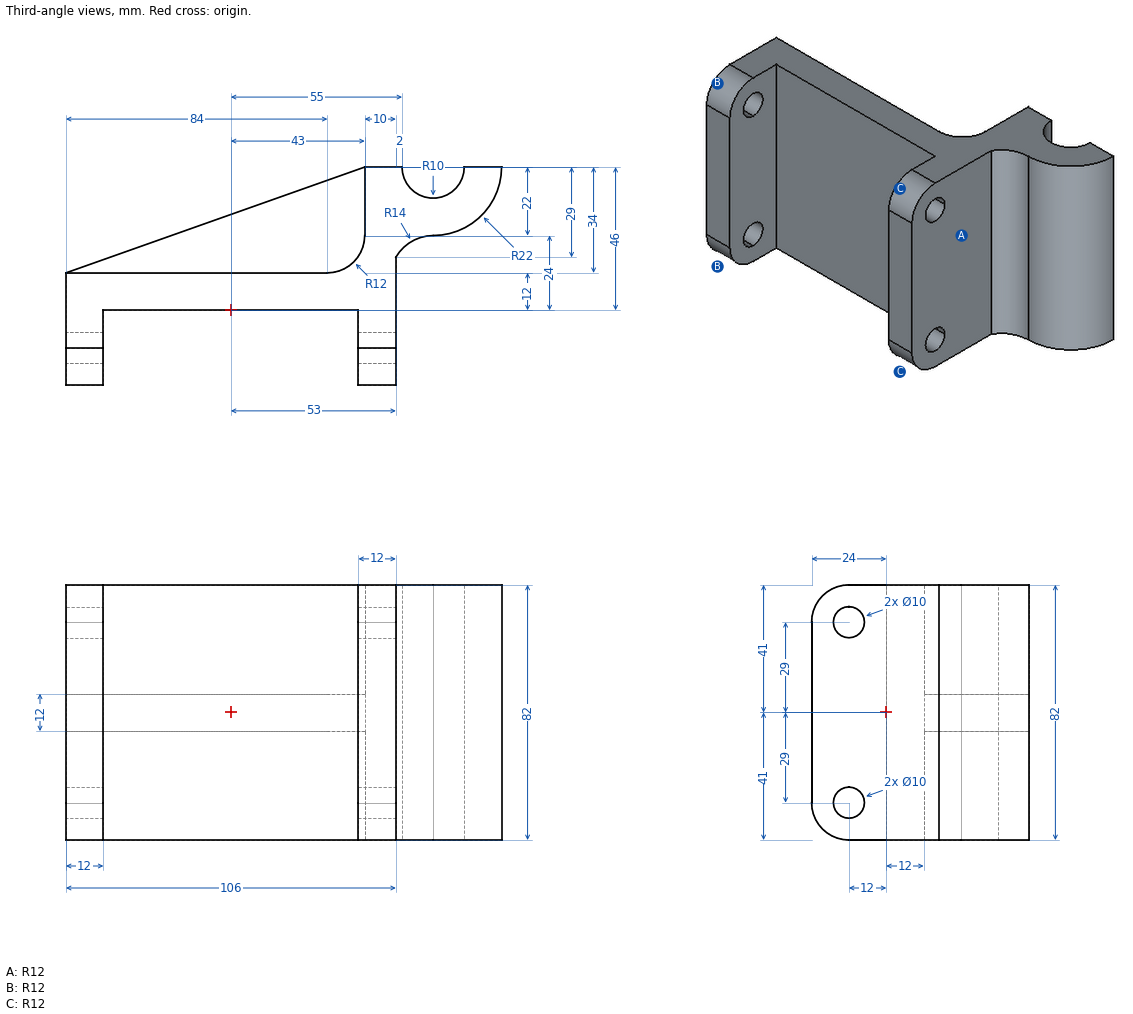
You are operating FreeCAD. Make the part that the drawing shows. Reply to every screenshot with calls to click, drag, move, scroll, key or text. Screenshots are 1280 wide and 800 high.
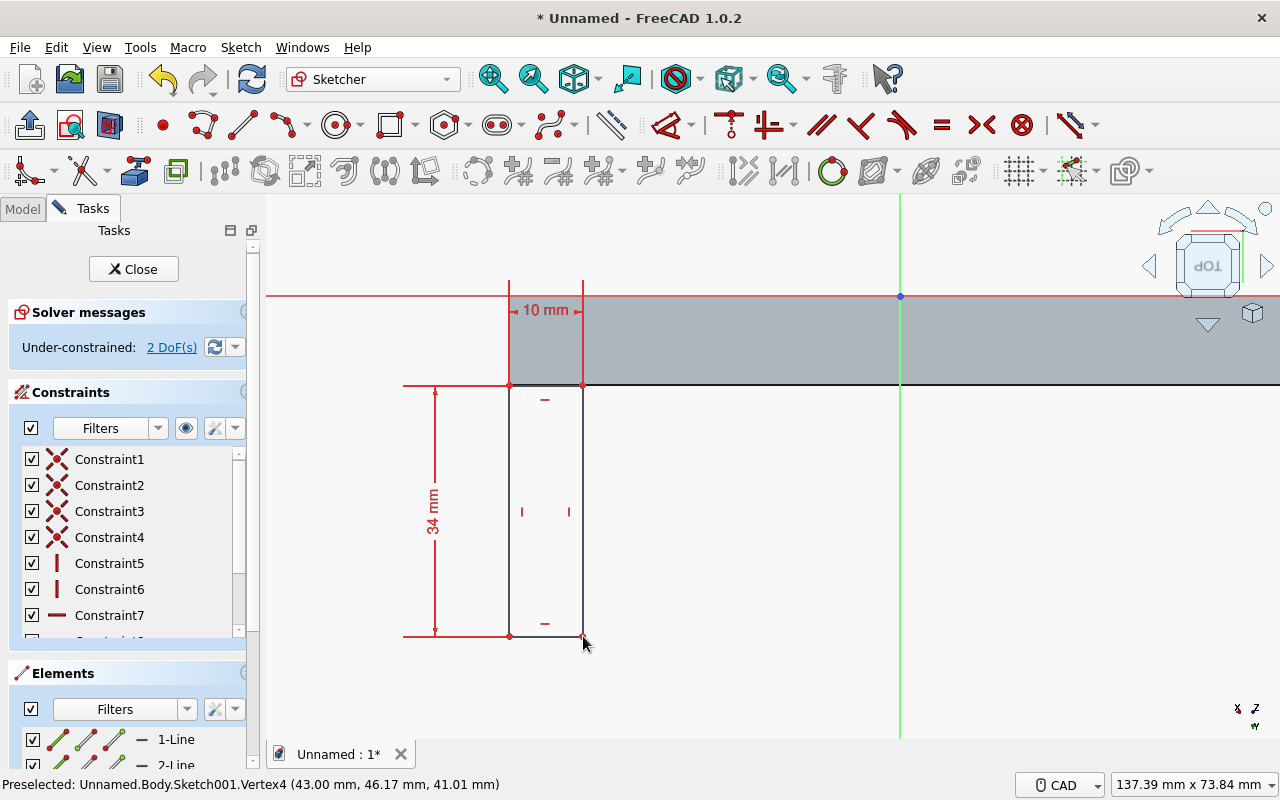
key(d)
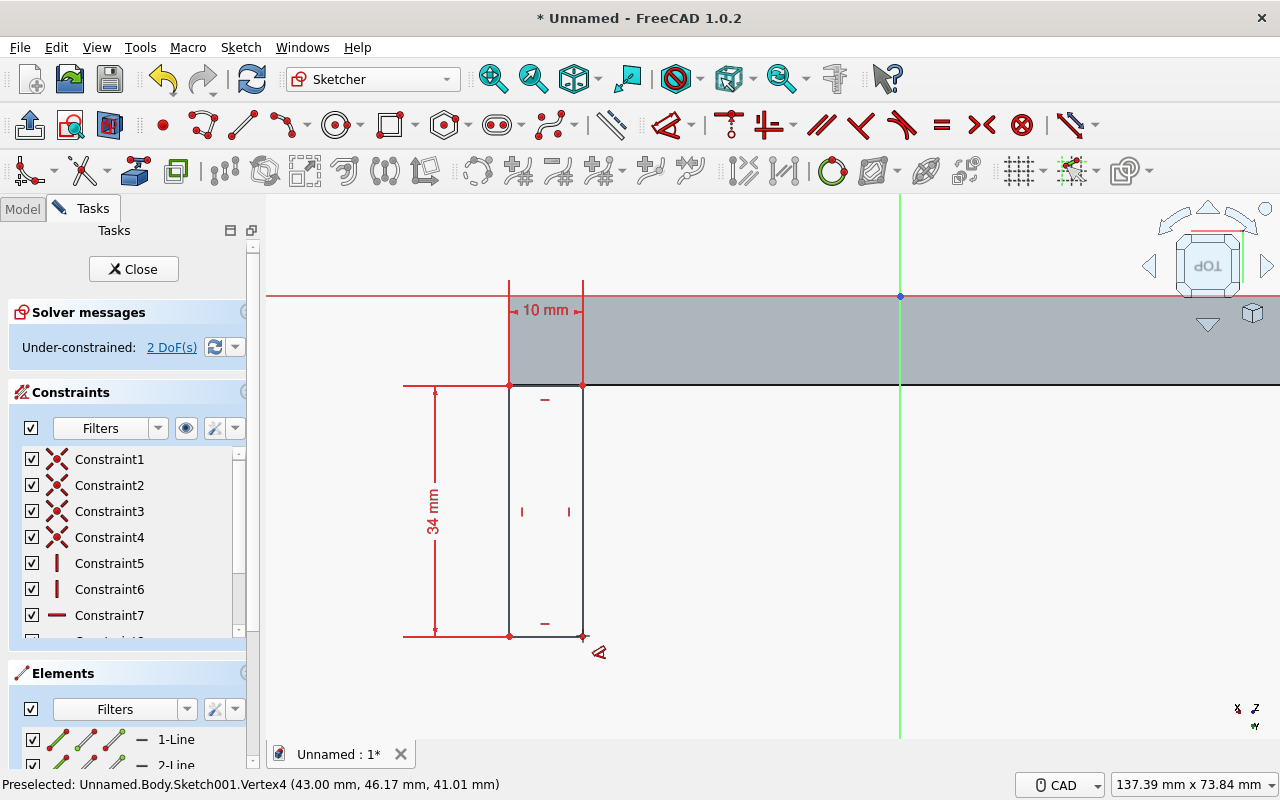
click(509, 386)
click(705, 262)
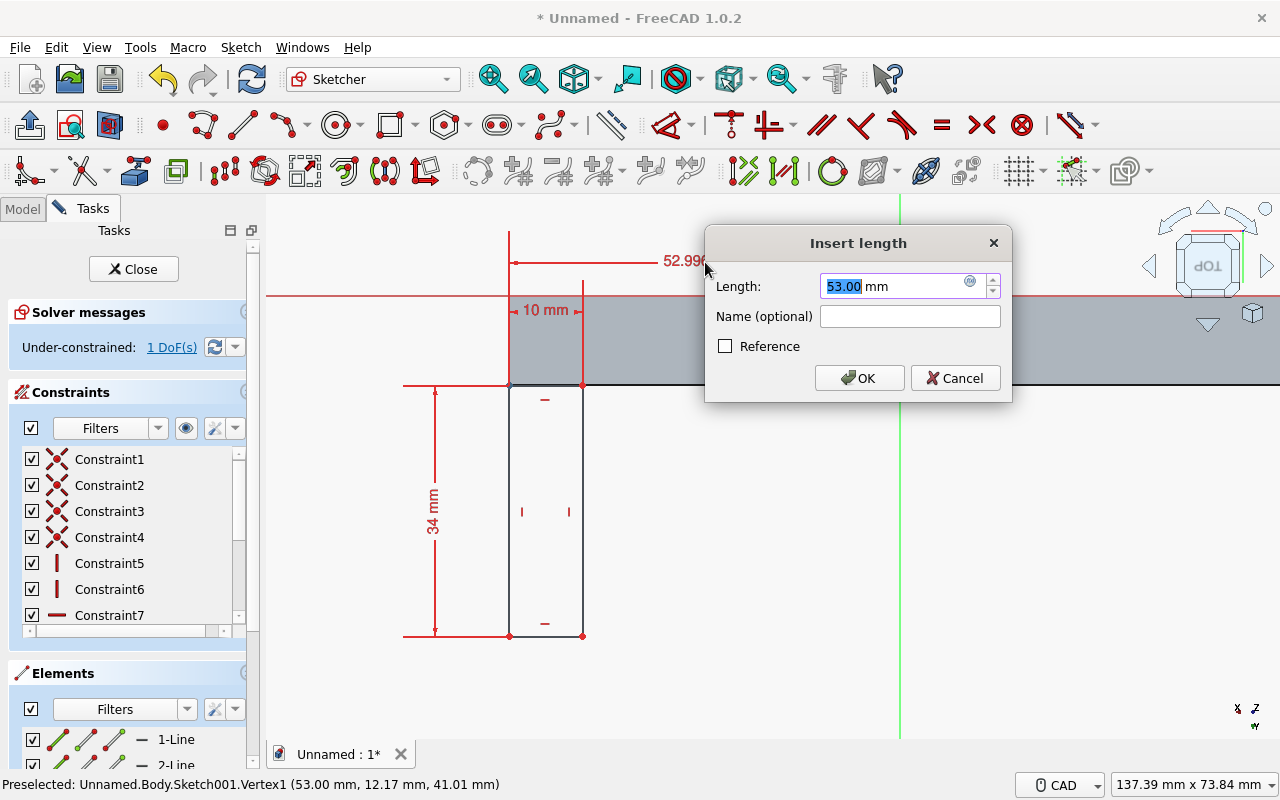
text(53)
key(Return)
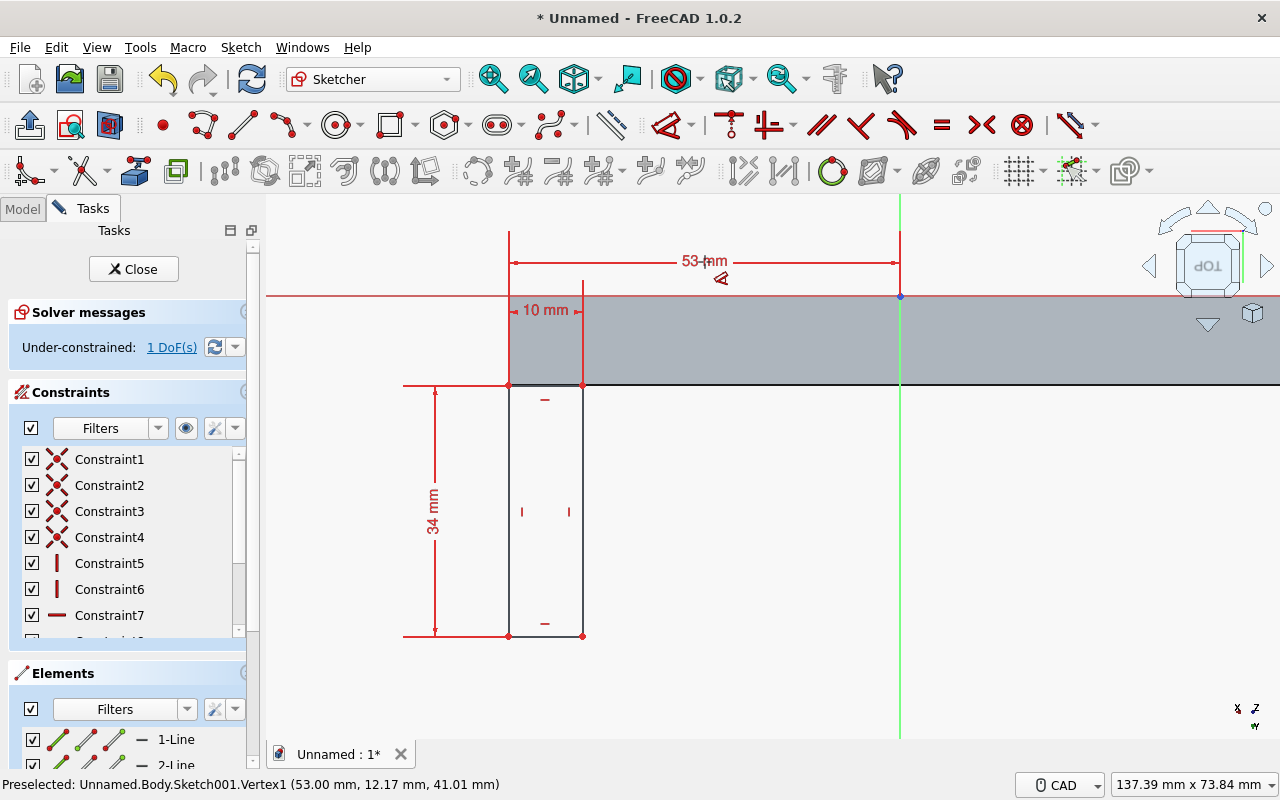
click(509, 386)
click(934, 341)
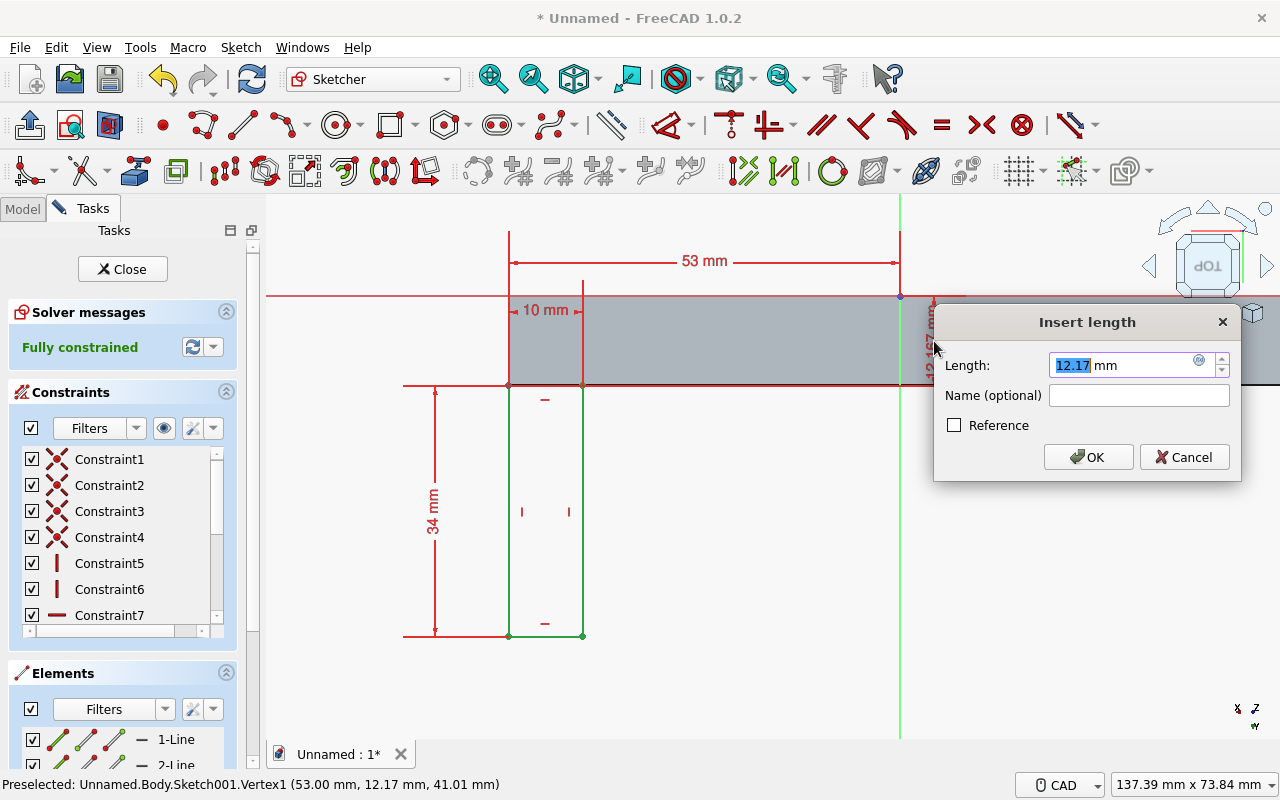
text(12)
key(Return)
key(Escape)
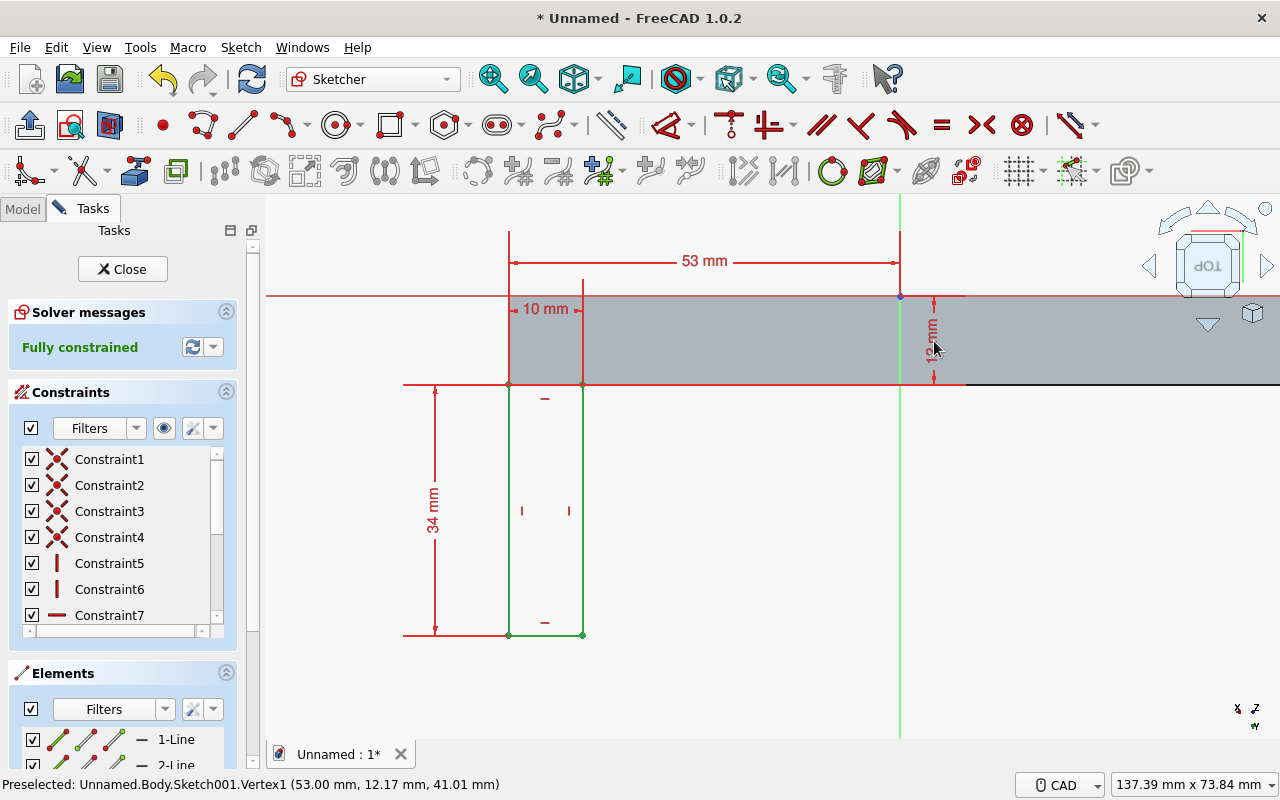
click(123, 269)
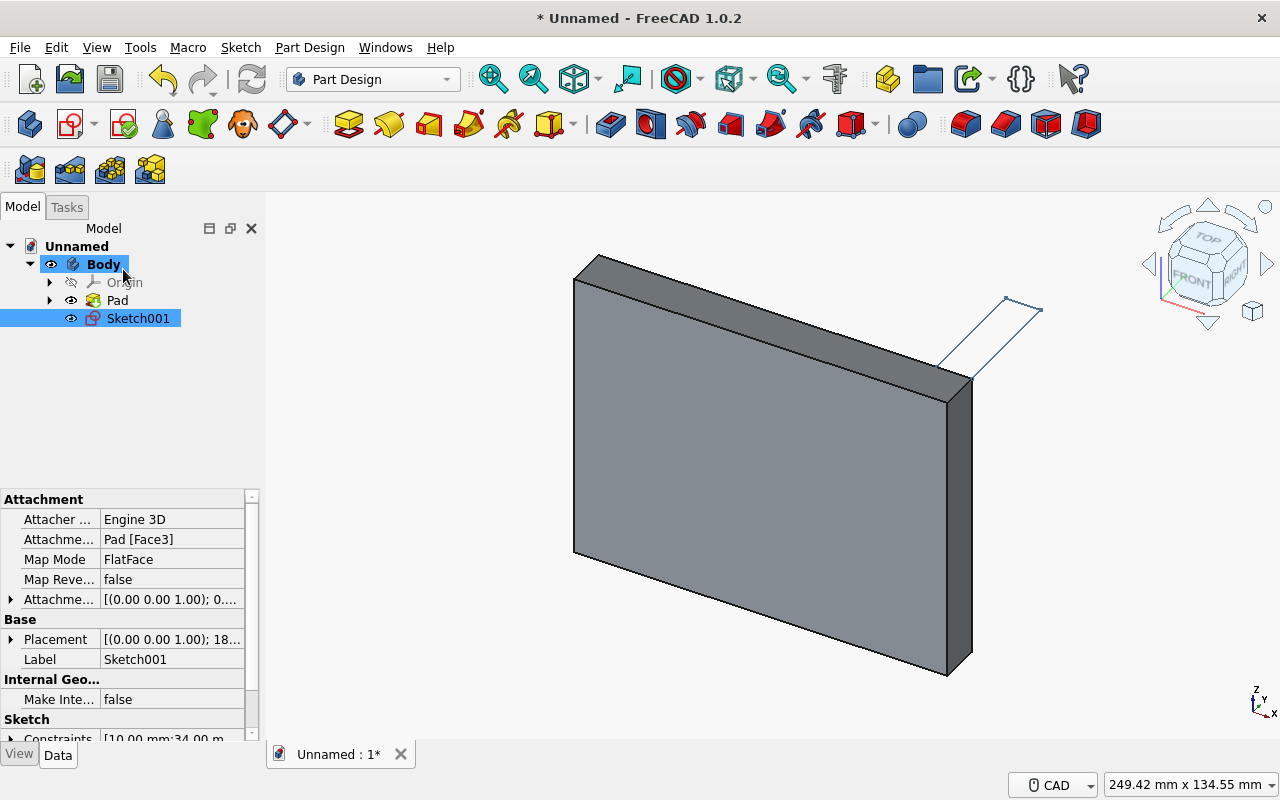
click(350, 124)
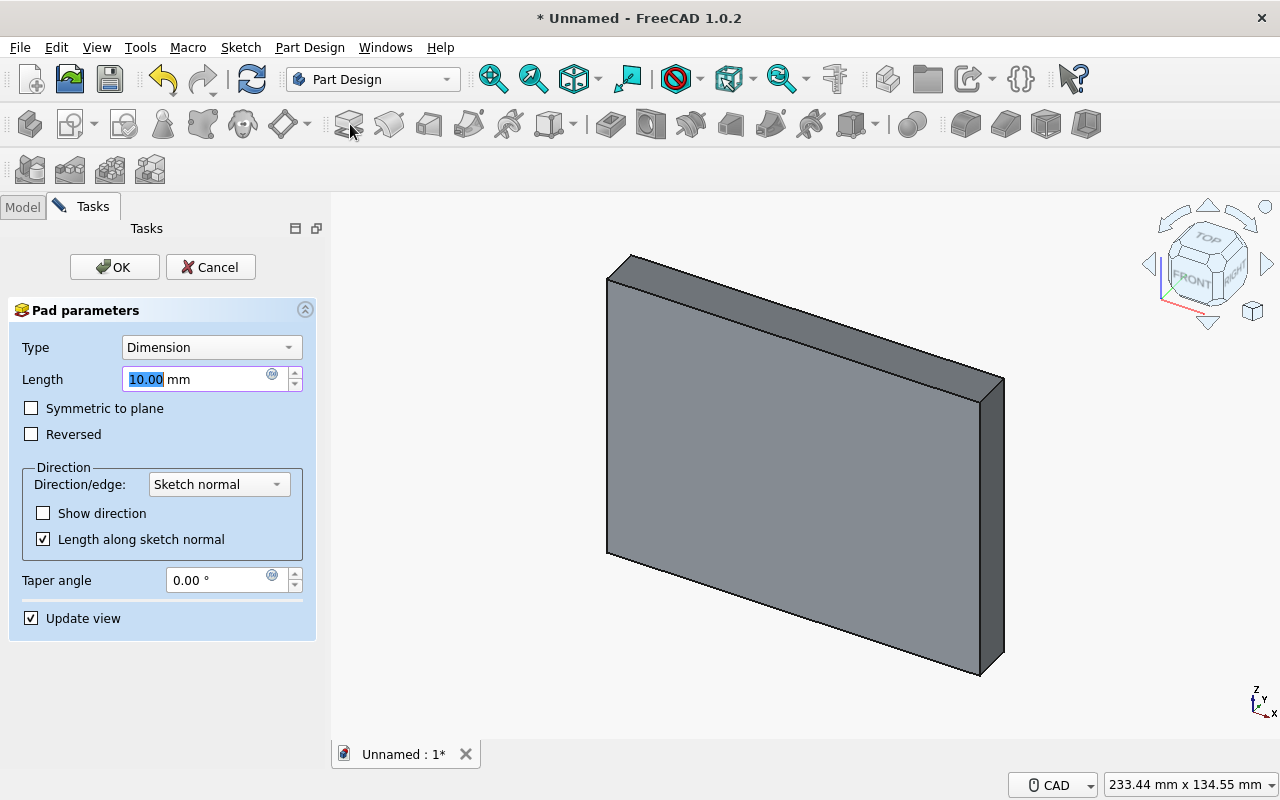
text(82)
key(Tab)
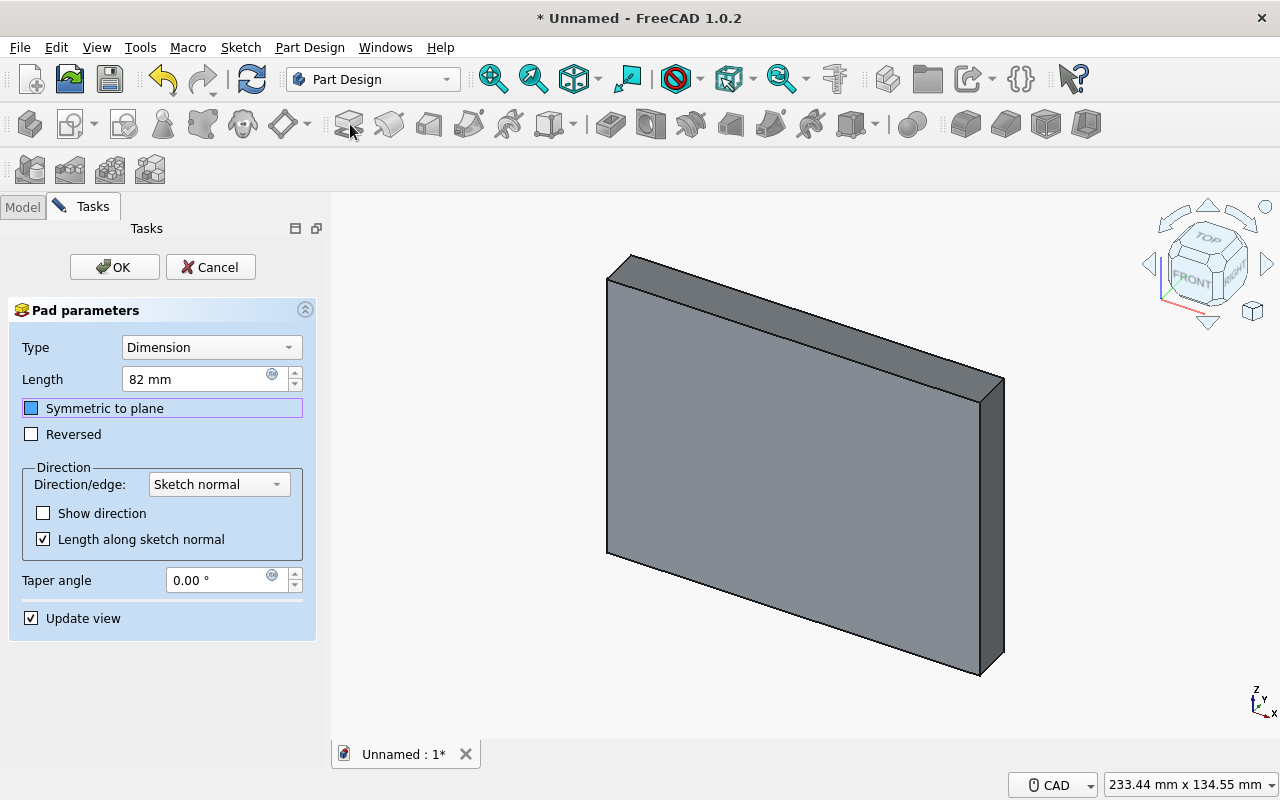
click(30, 434)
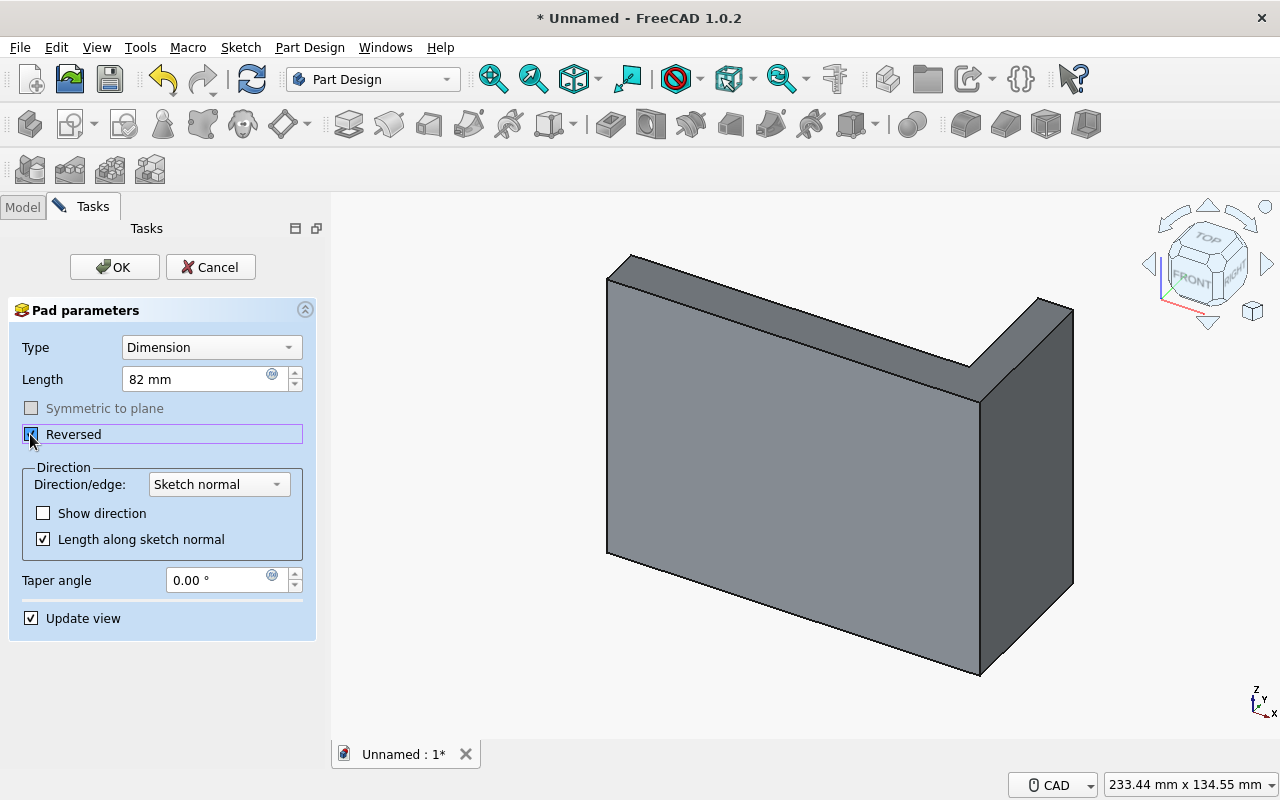
click(115, 267)